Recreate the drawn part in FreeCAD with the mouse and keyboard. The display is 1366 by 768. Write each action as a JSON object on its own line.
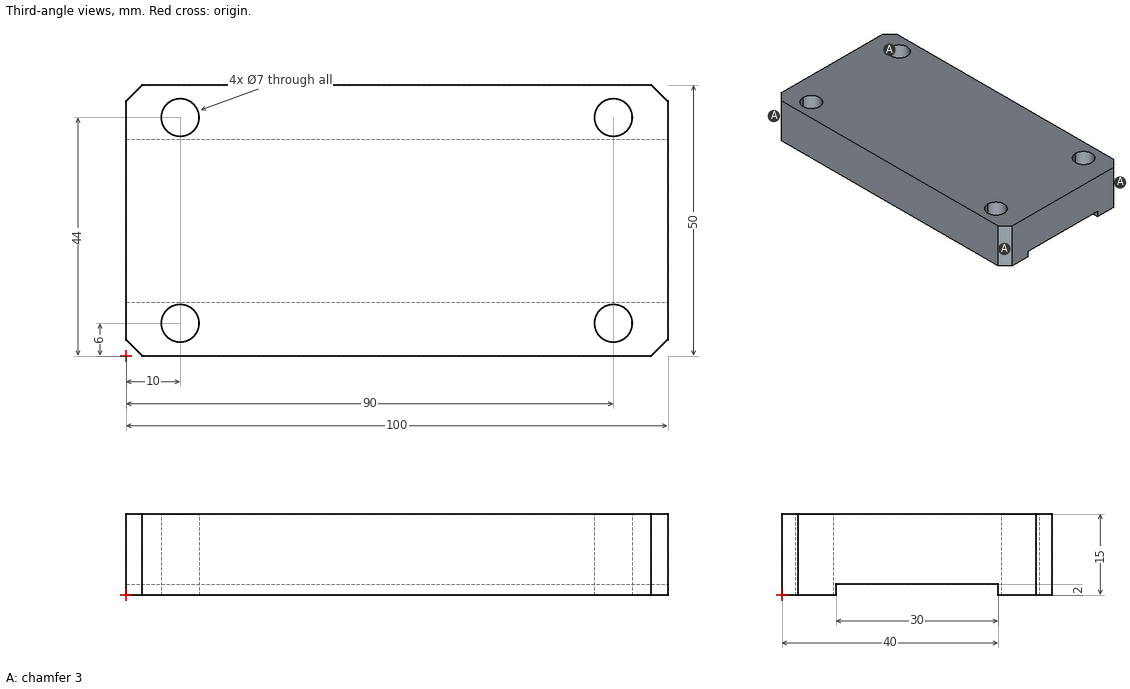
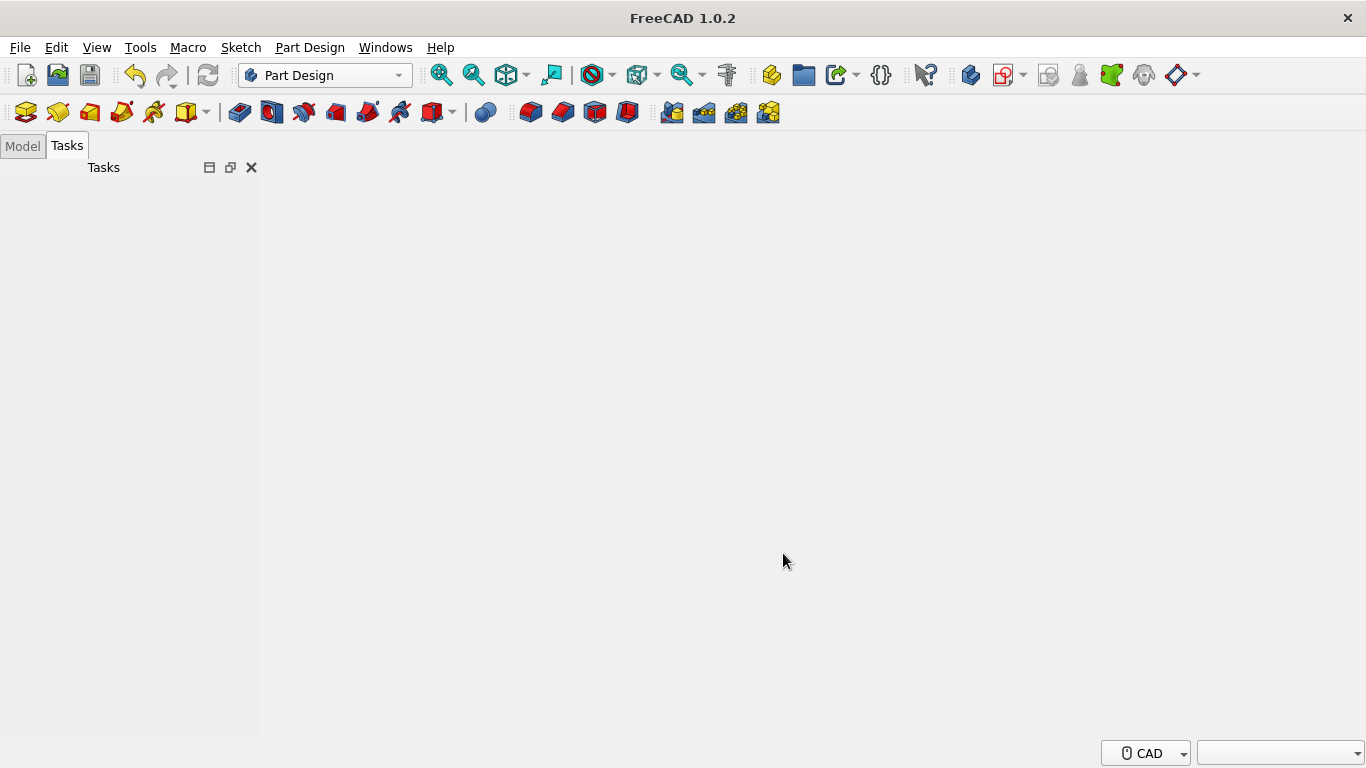
{"action": "key", "text": "ctrl+n"}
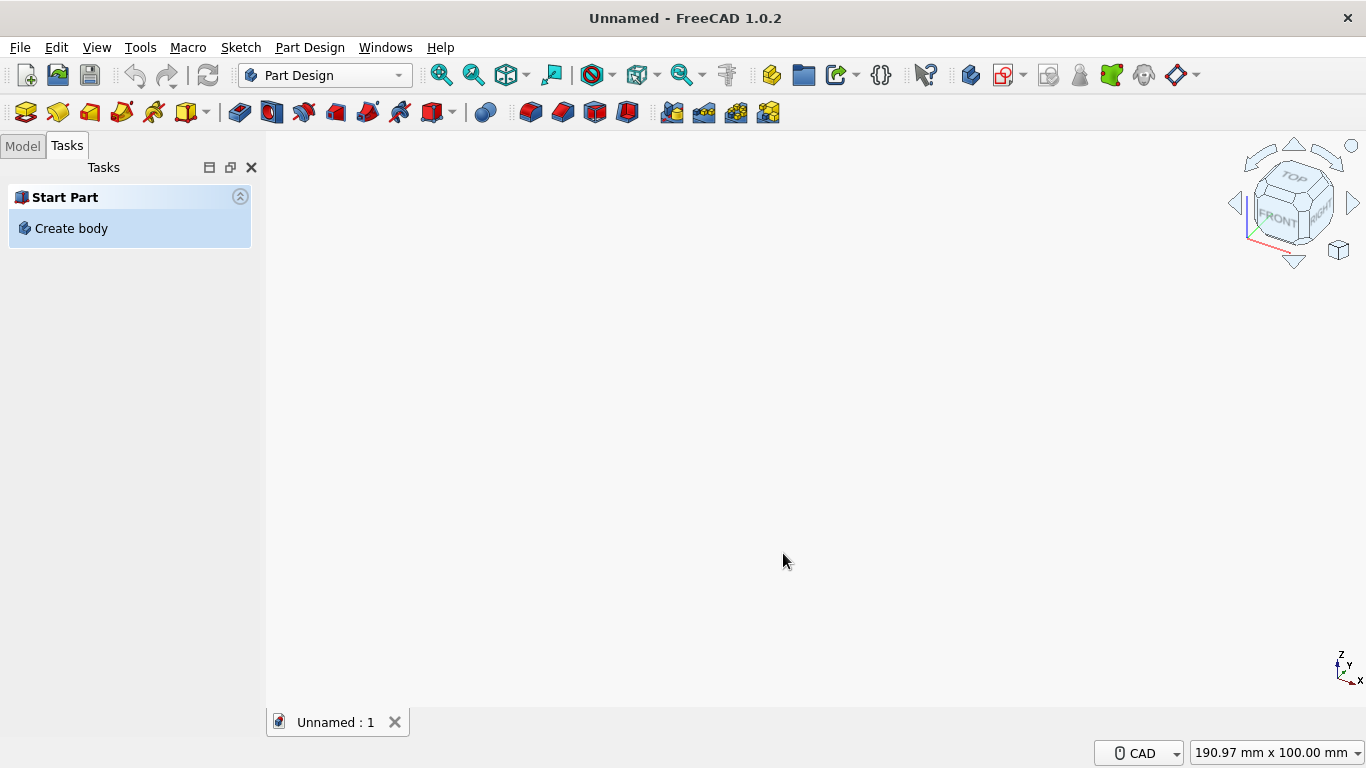
{"action": "left_click", "coordinate": [1004, 76]}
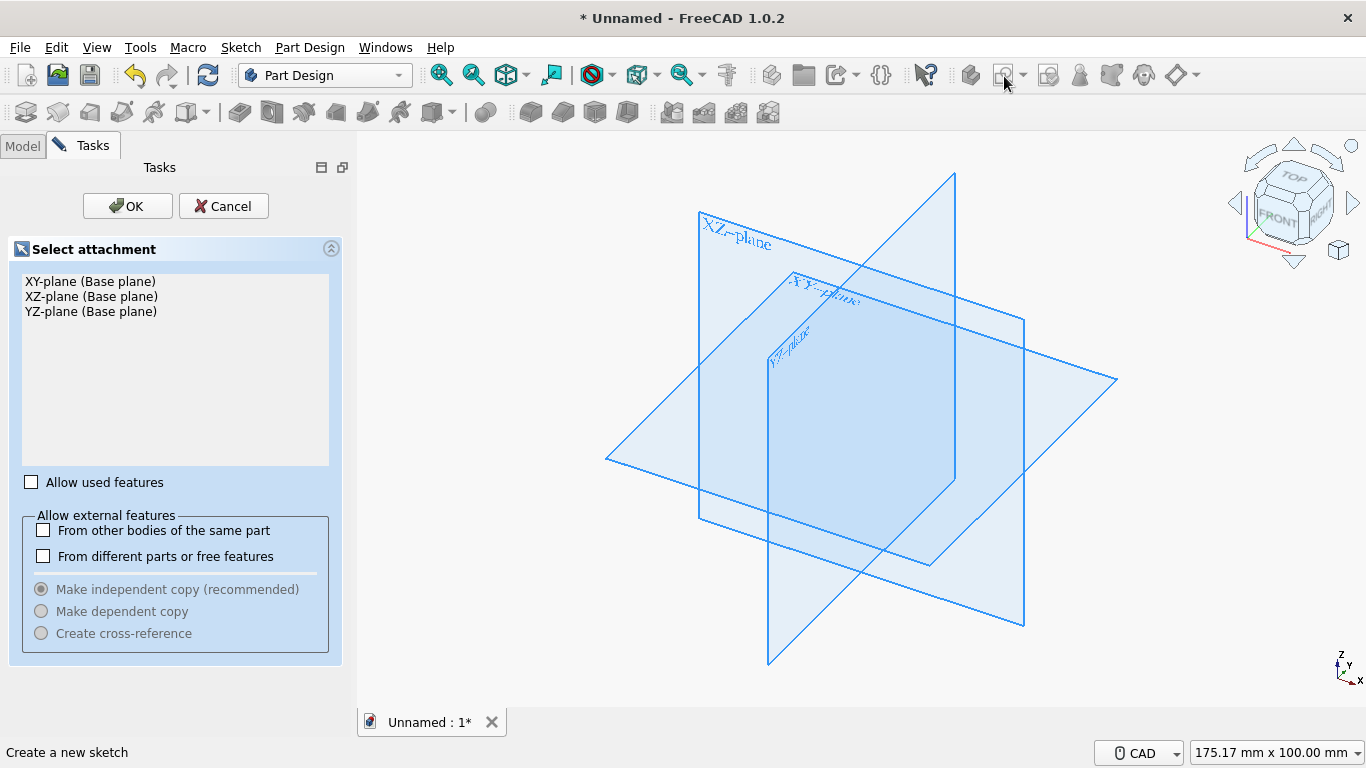
{"action": "left_click", "coordinate": [82, 282]}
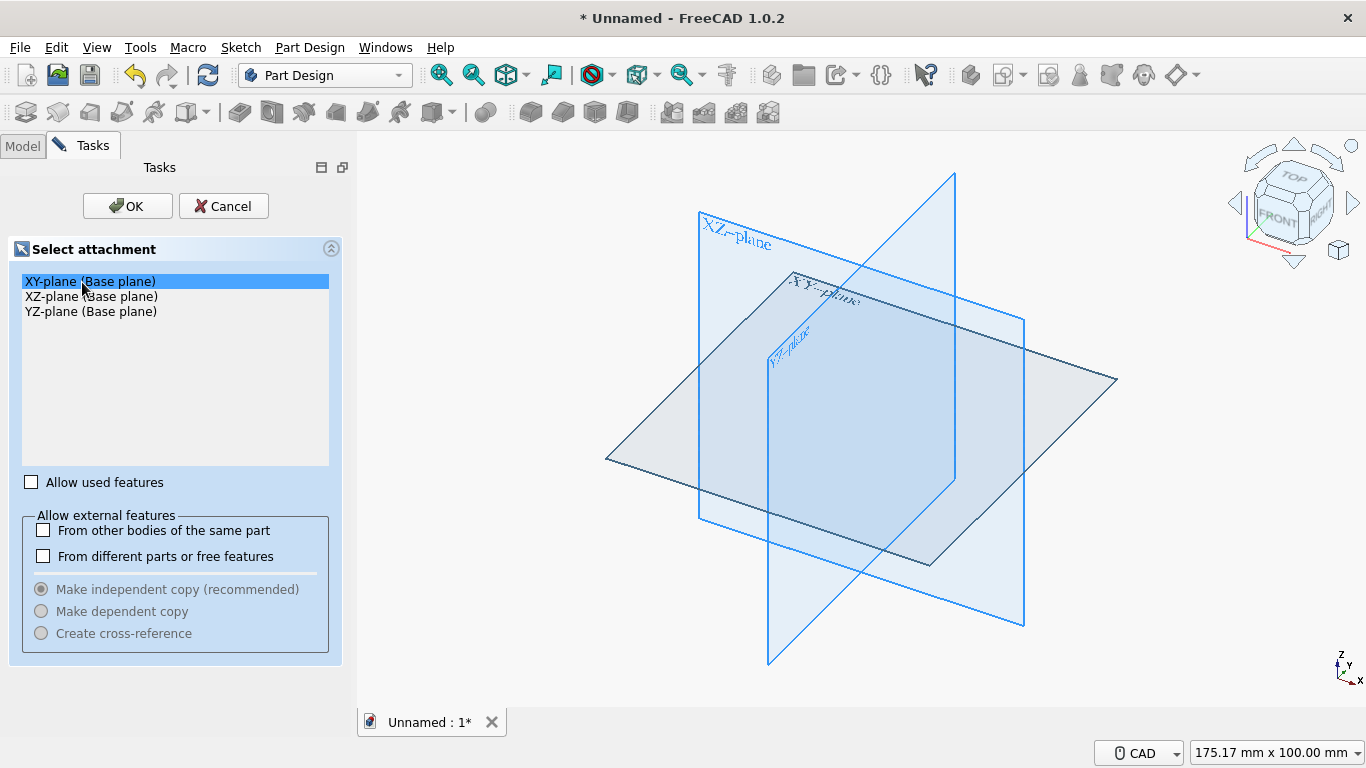
{"action": "left_click", "coordinate": [128, 206]}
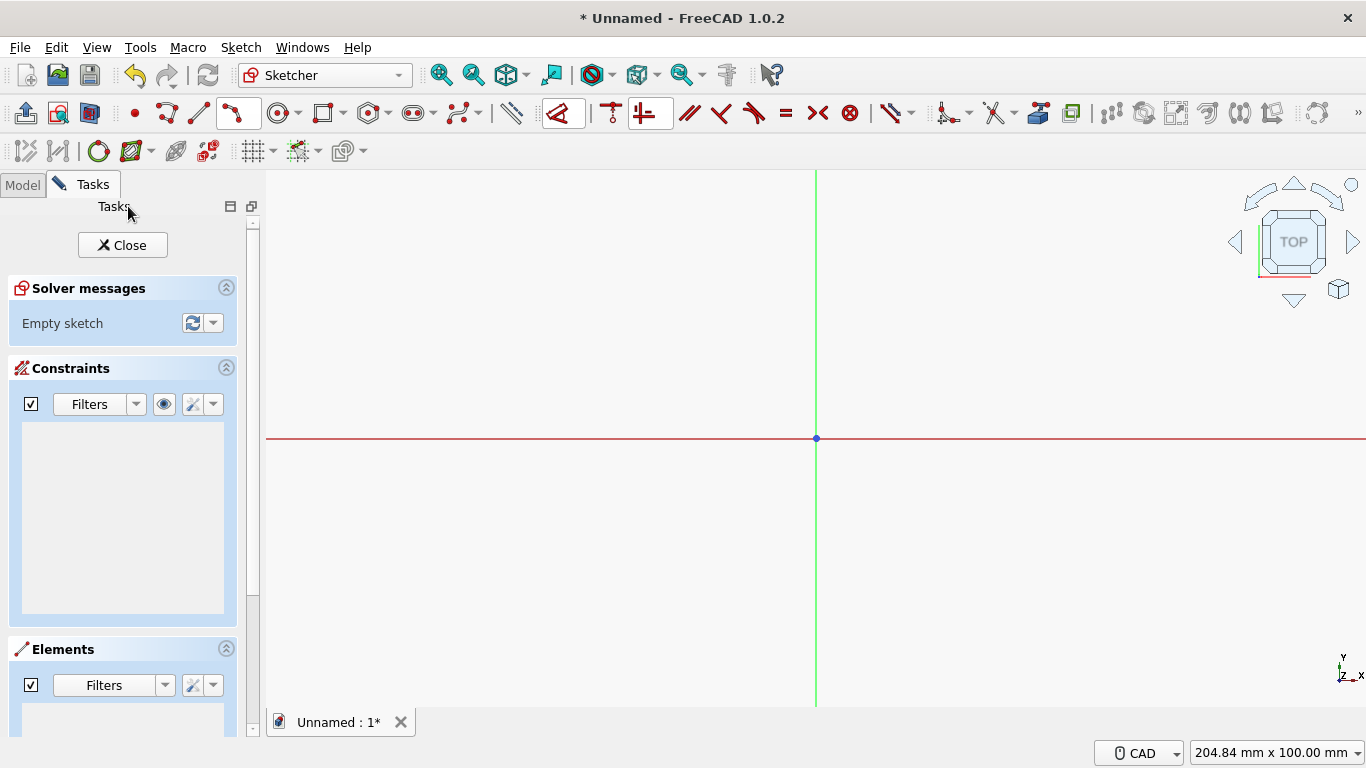
{"action": "scroll", "coordinate": [294, 679], "scroll_direction": "down", "scroll_amount": 1}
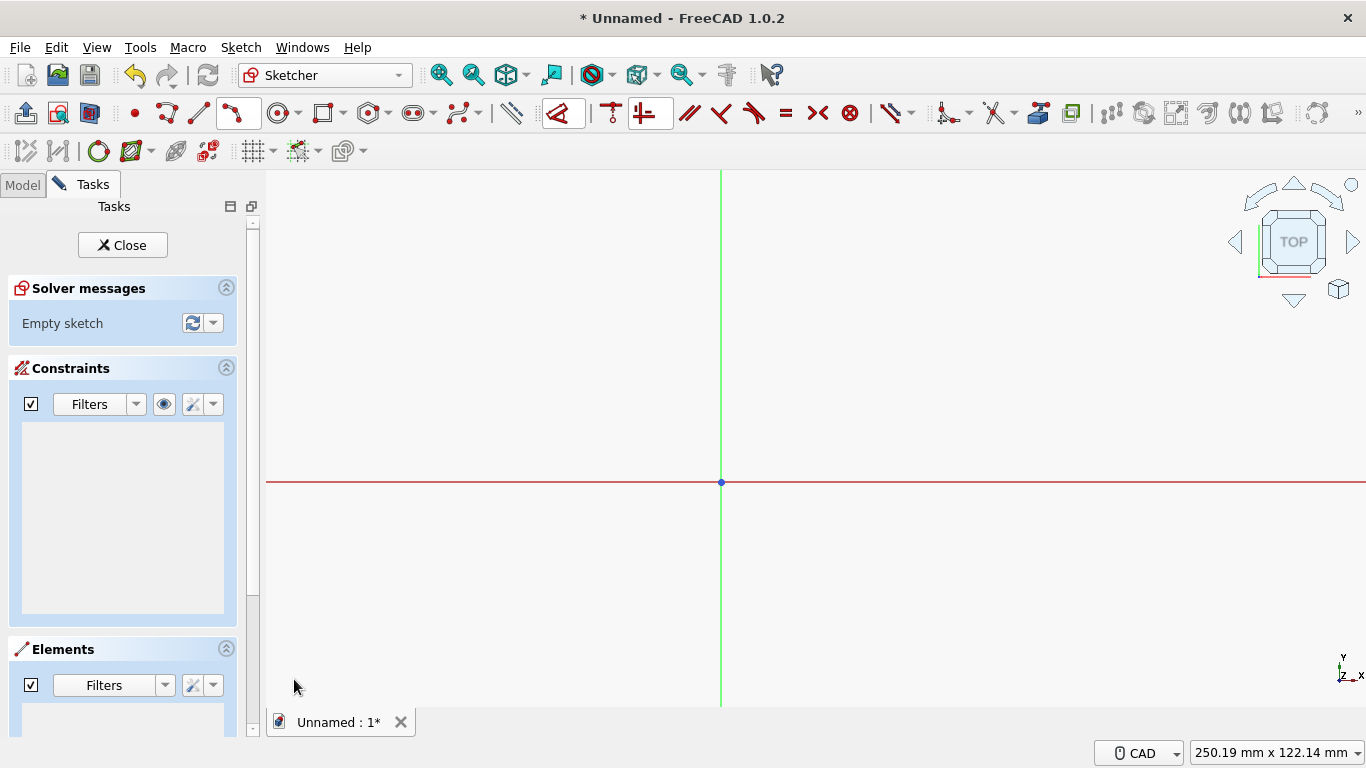
{"action": "scroll", "coordinate": [1201, 238], "scroll_direction": "up", "scroll_amount": 2}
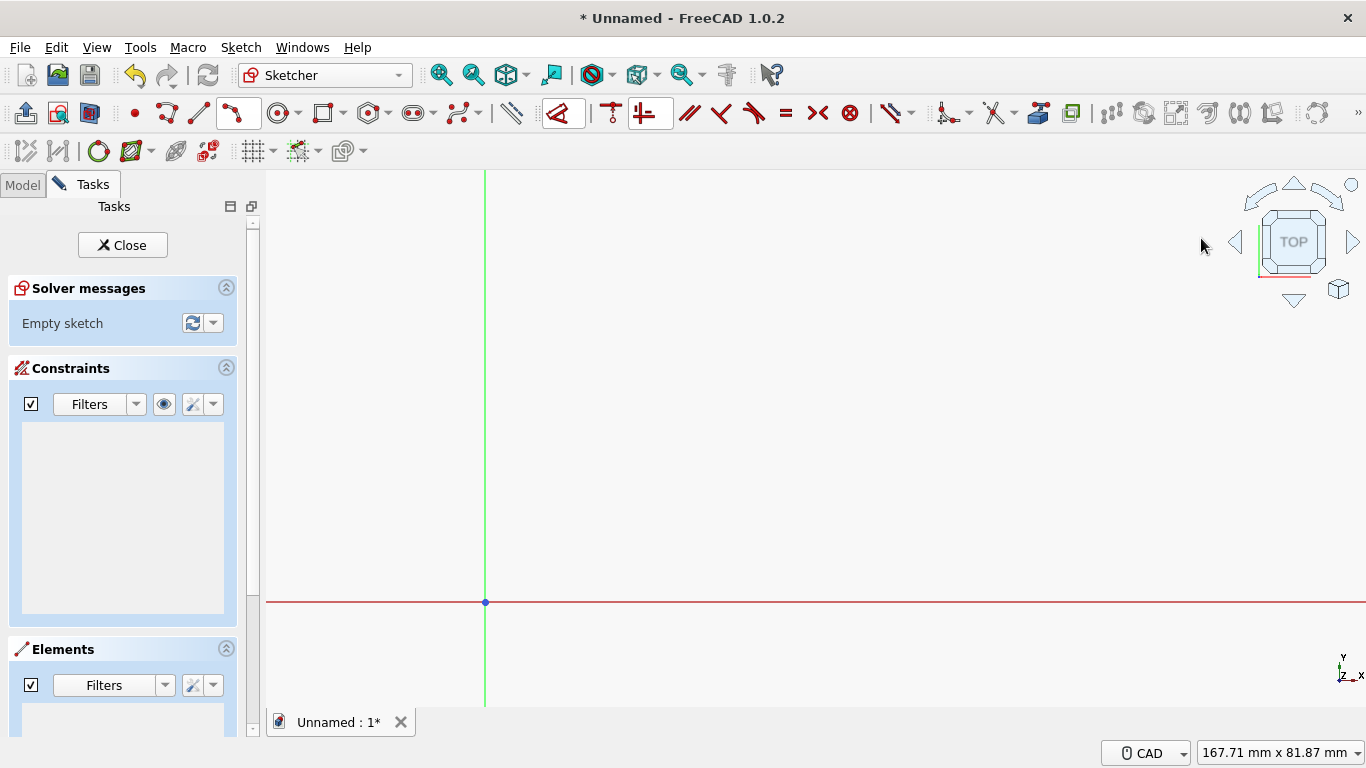
{"action": "left_click", "coordinate": [324, 114]}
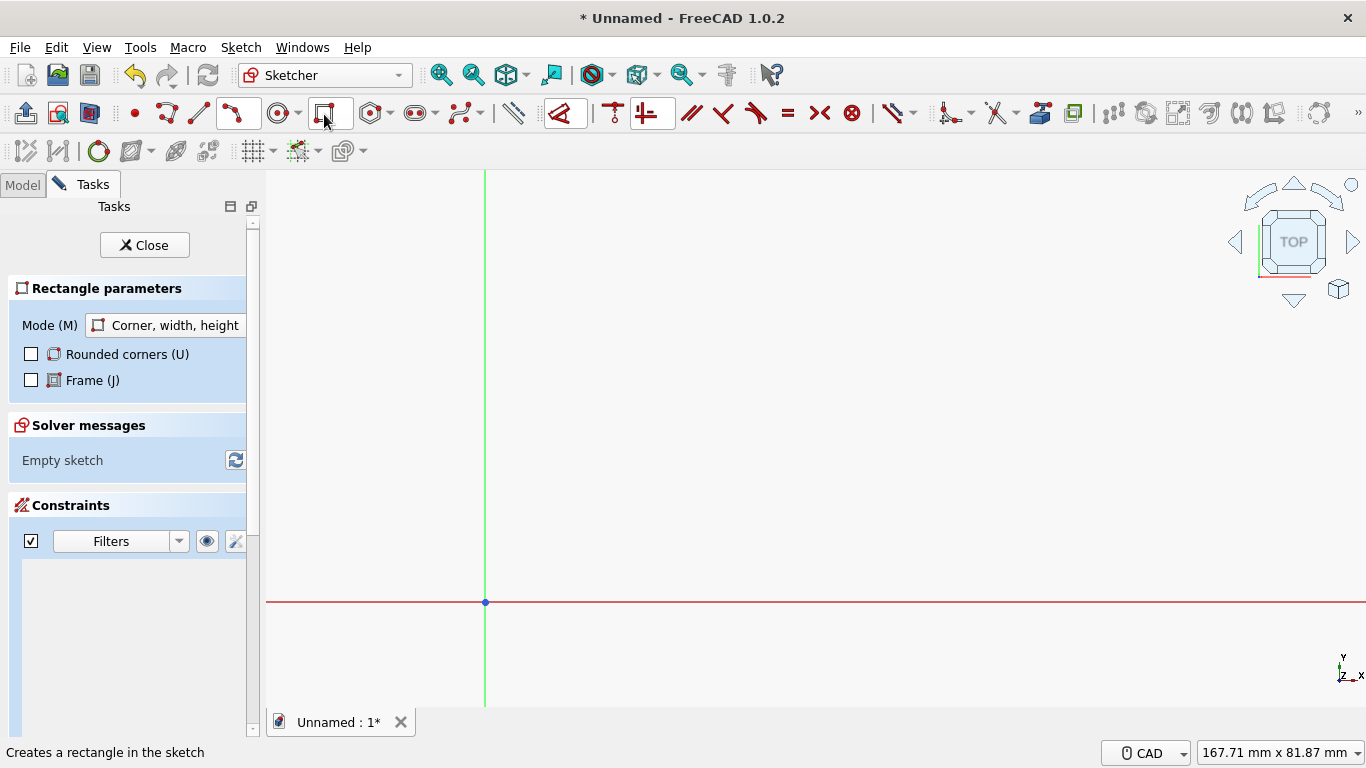
{"action": "left_click", "coordinate": [485, 602]}
{"action": "mouse_move", "coordinate": [1141, 274]}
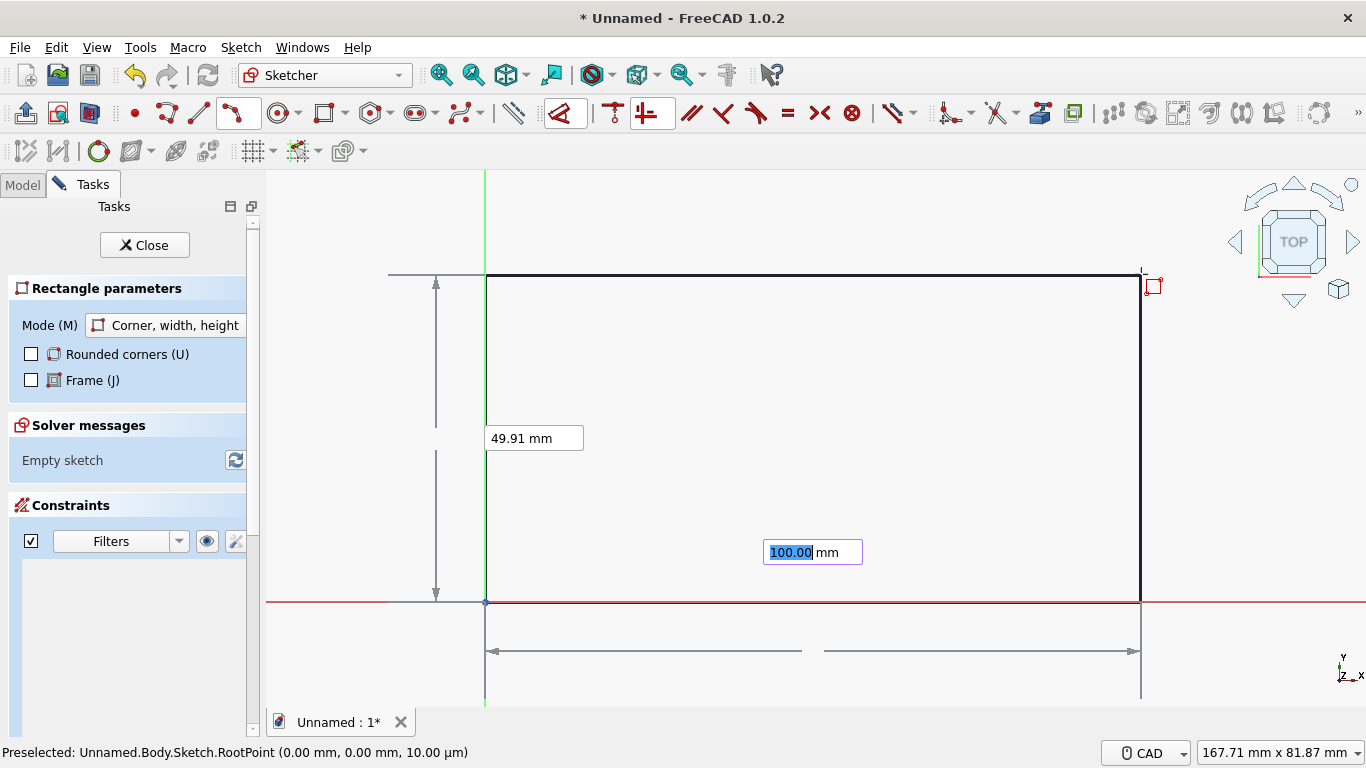
{"action": "type", "text": "100"}
{"action": "key", "text": "Tab"}
{"action": "type", "text": "50"}
{"action": "key", "text": "Return"}
{"action": "key", "text": "Escape"}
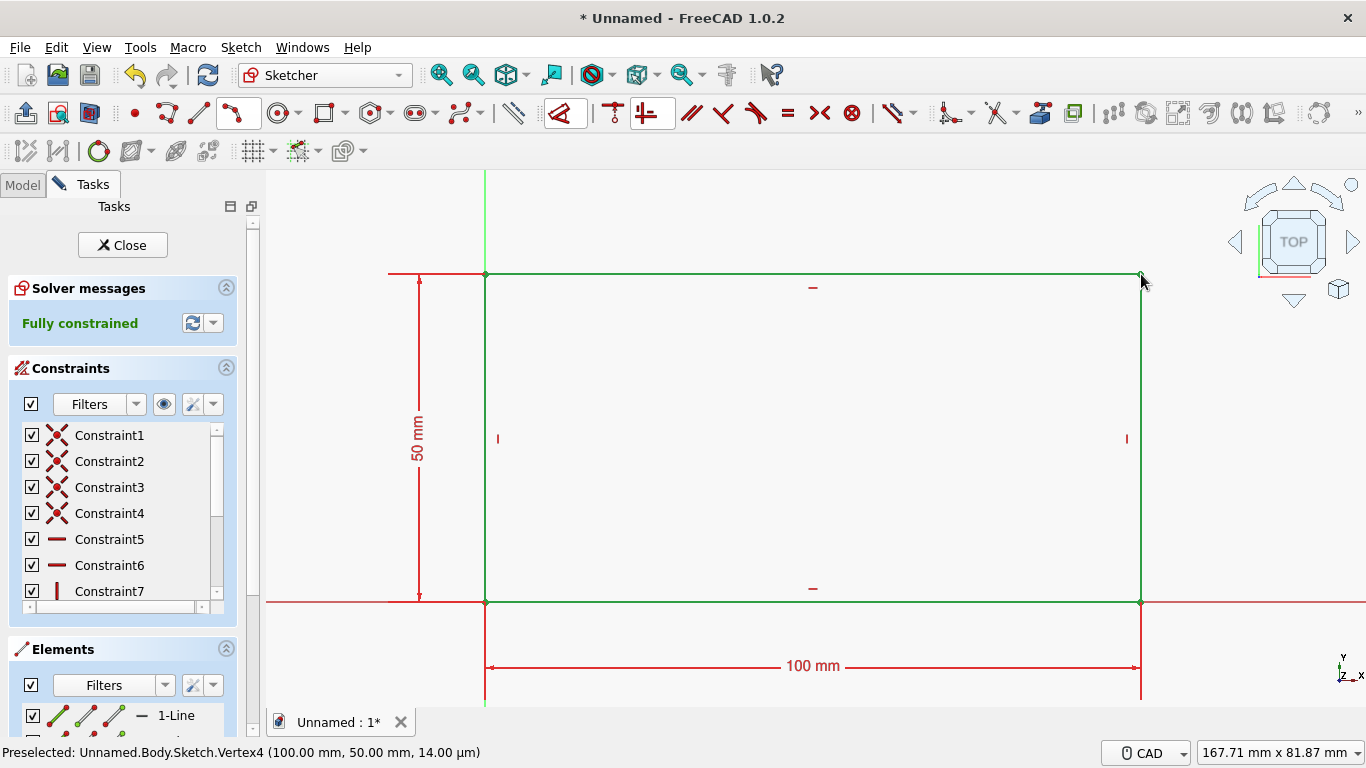
{"action": "left_click", "coordinate": [123, 245]}